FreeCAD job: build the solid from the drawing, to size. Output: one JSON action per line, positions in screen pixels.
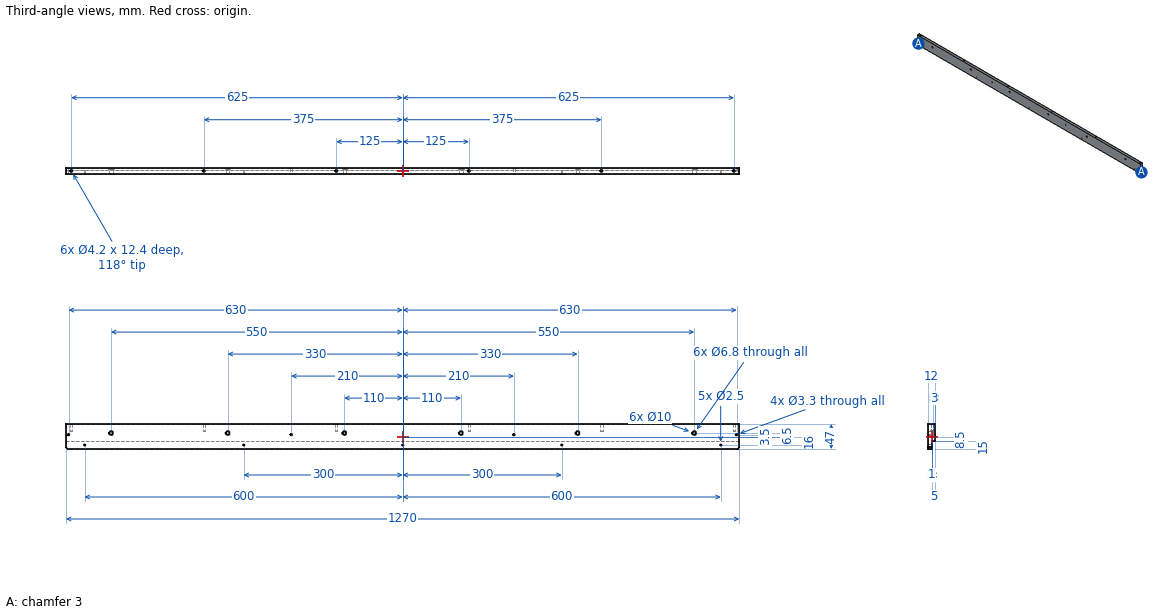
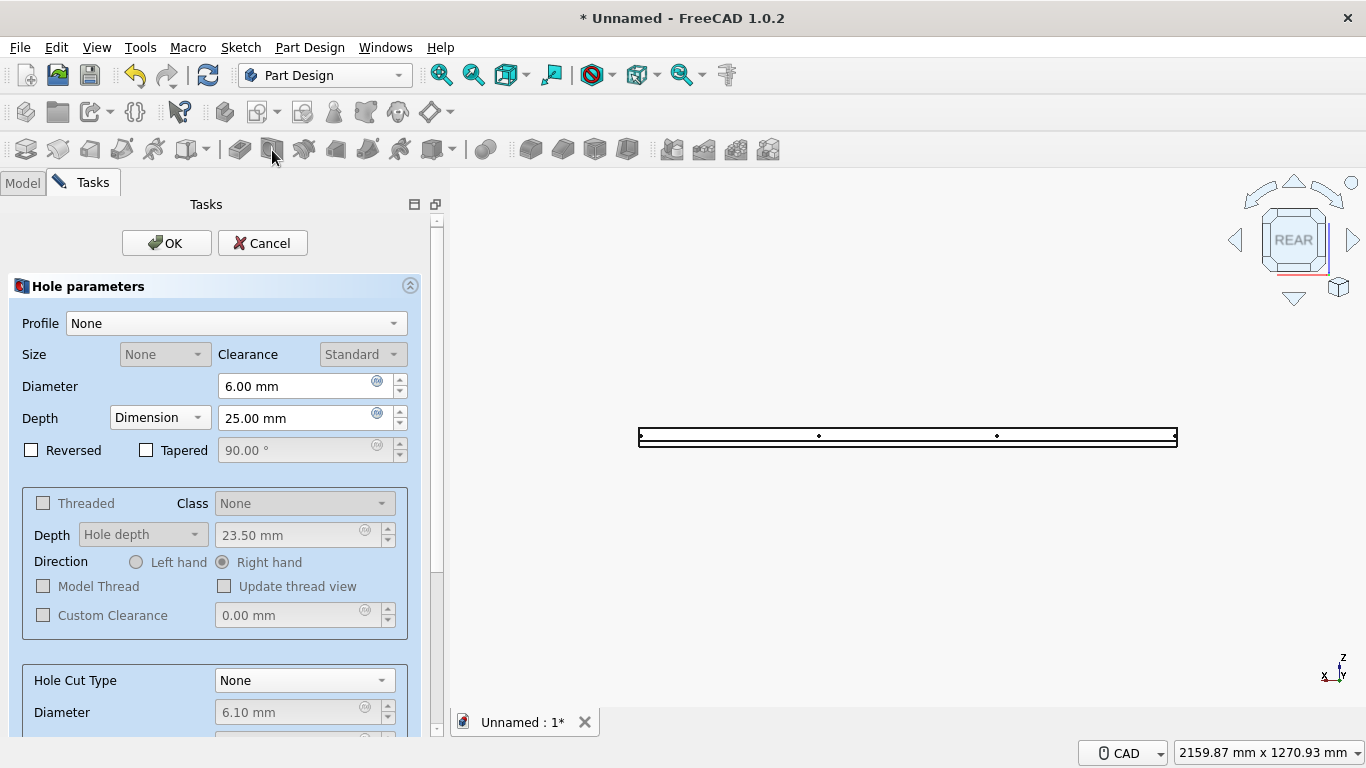
{"action": "triple_click", "coordinate": [305, 386]}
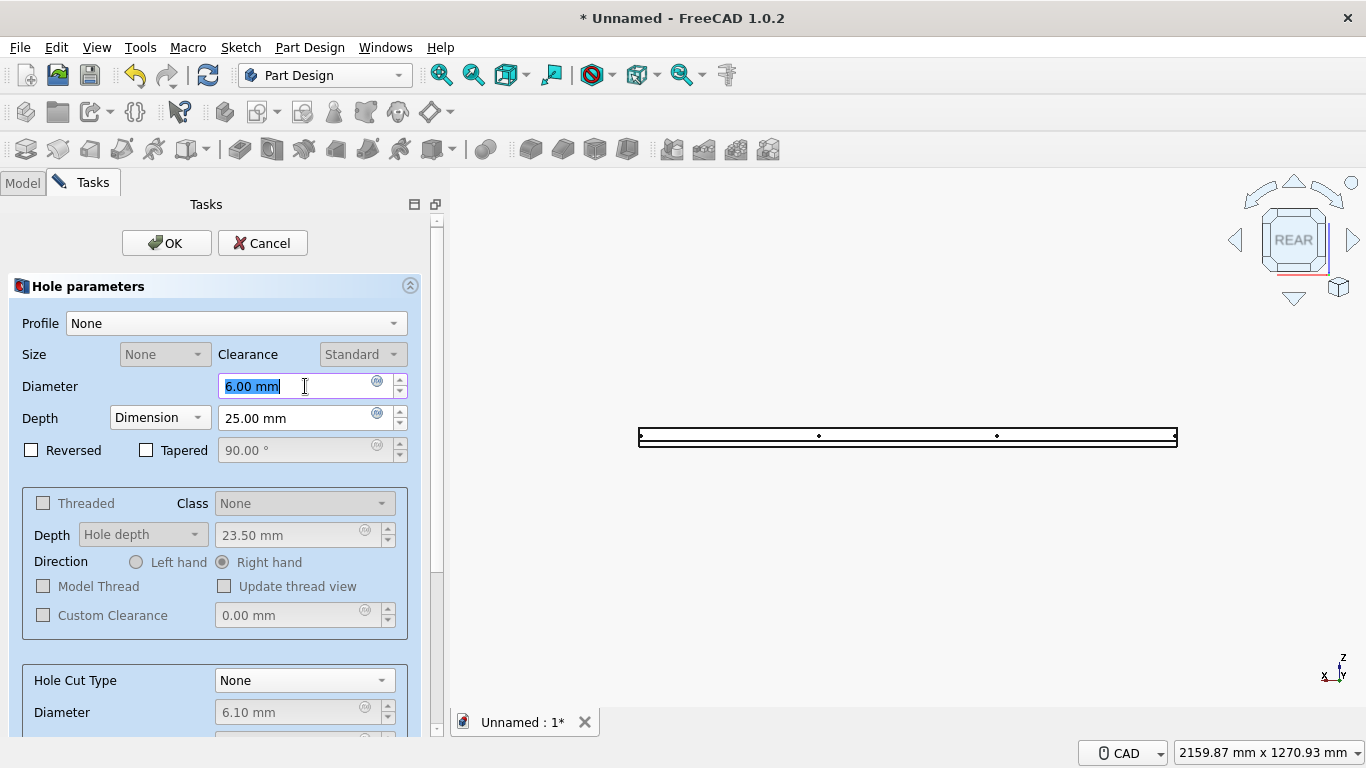
{"action": "type", "text": "3.3"}
{"action": "key", "text": "Tab"}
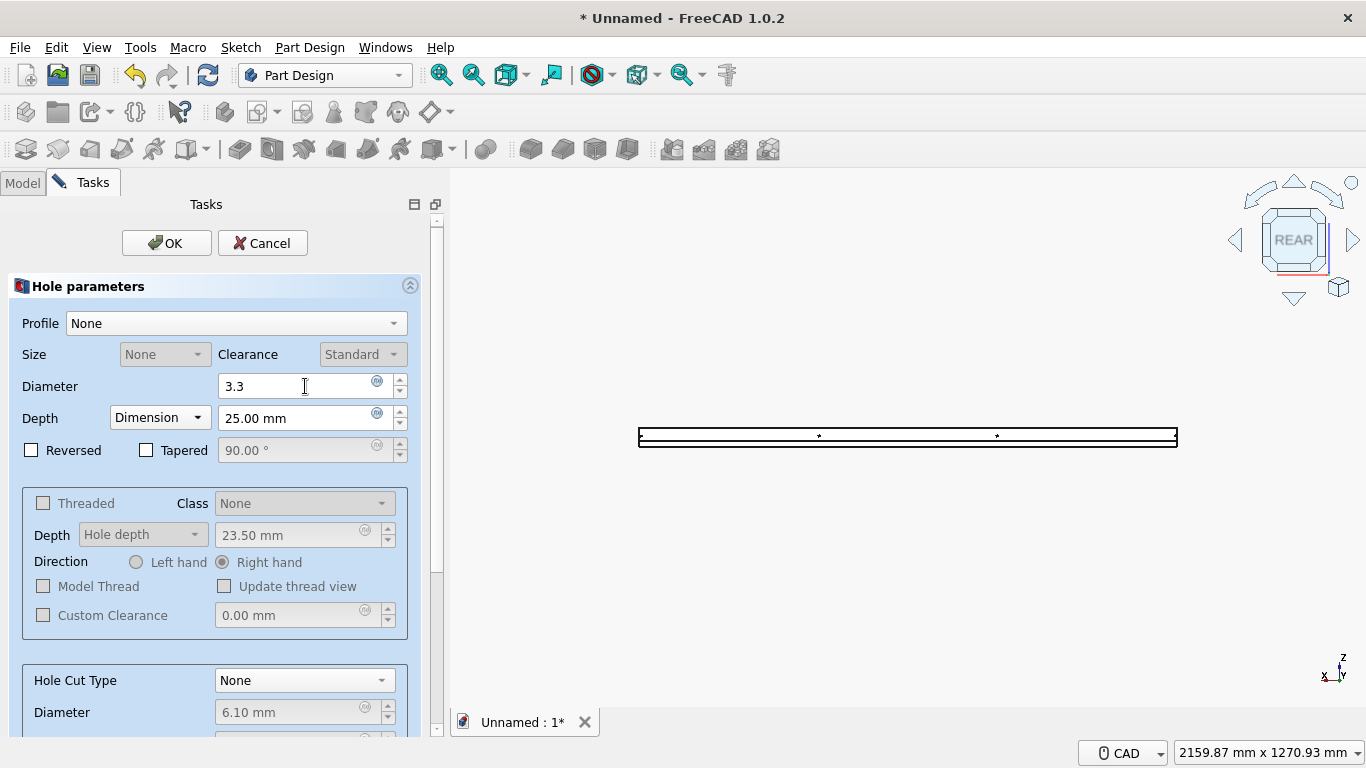
{"action": "left_click", "coordinate": [161, 418]}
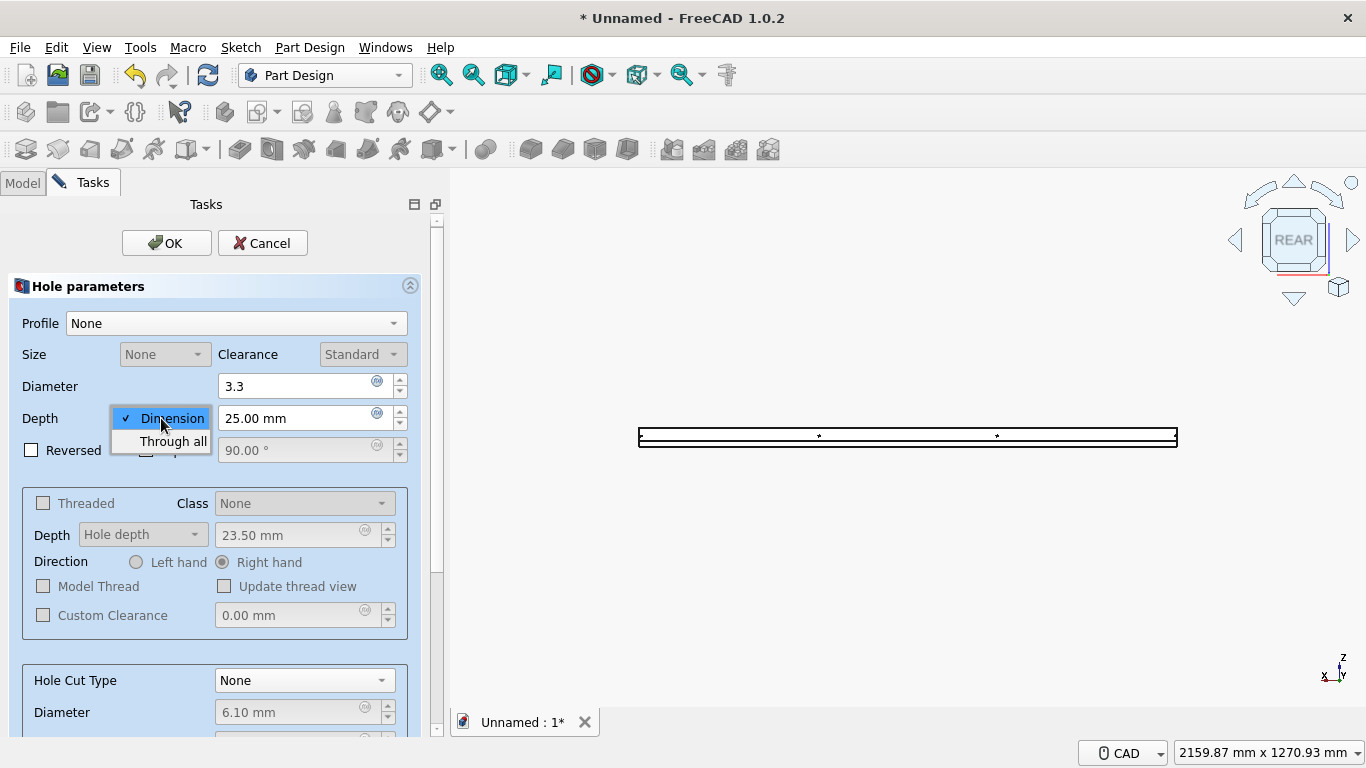
{"action": "left_click", "coordinate": [160, 442]}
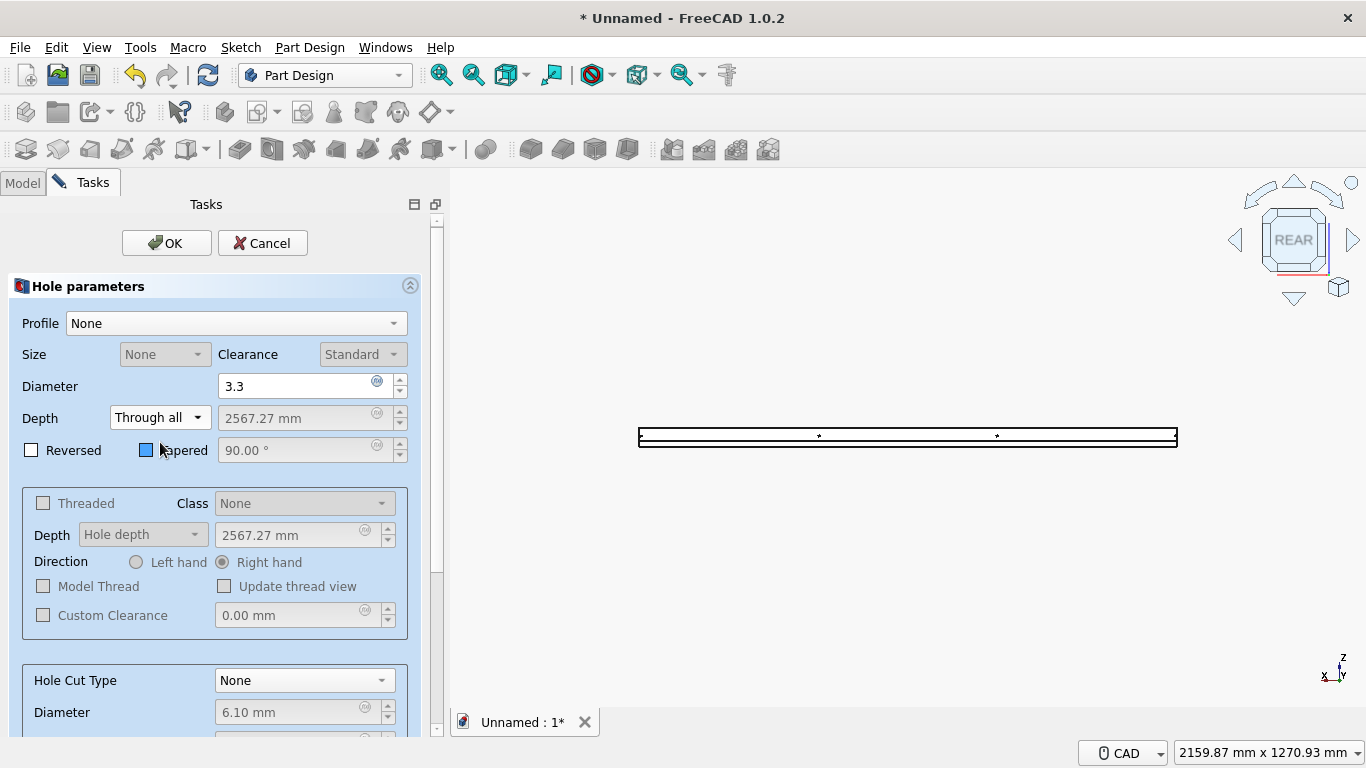
{"action": "left_click", "coordinate": [167, 243]}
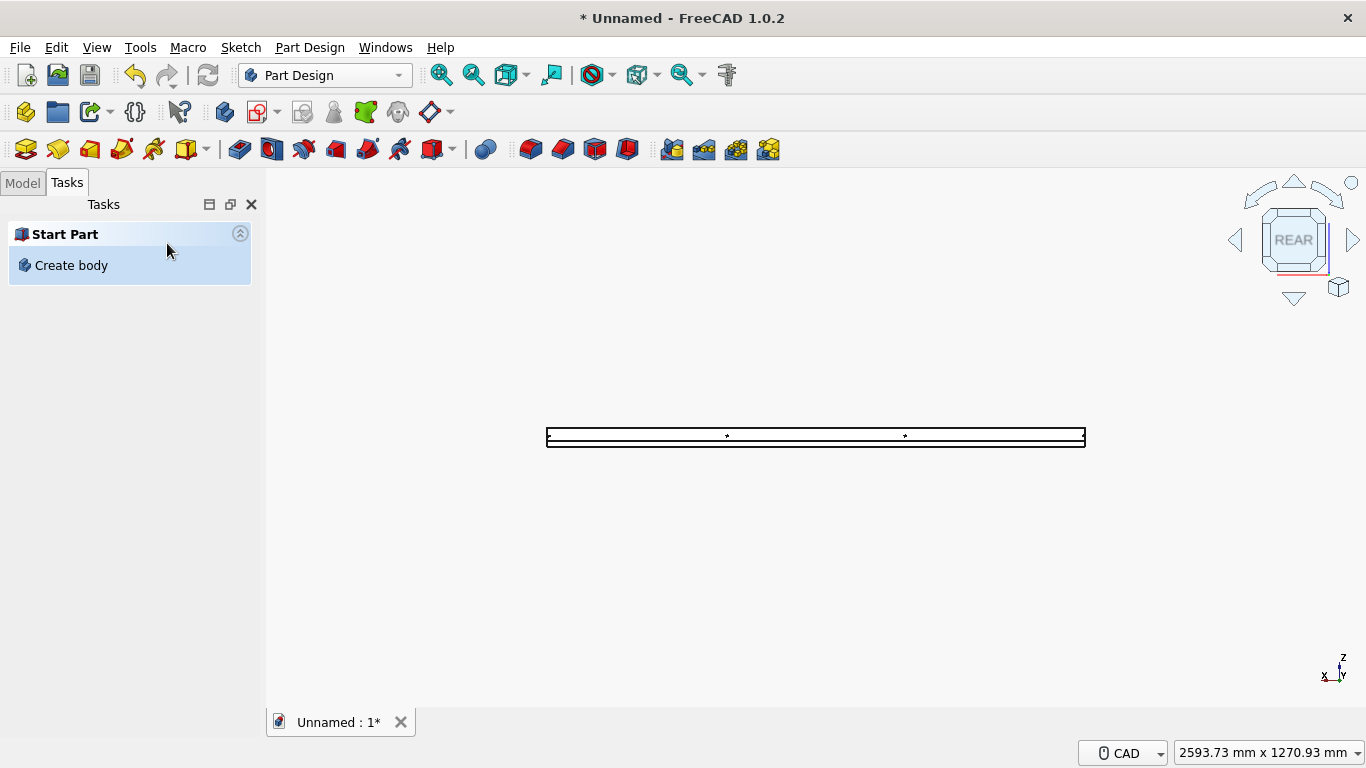
{"action": "key", "text": "0"}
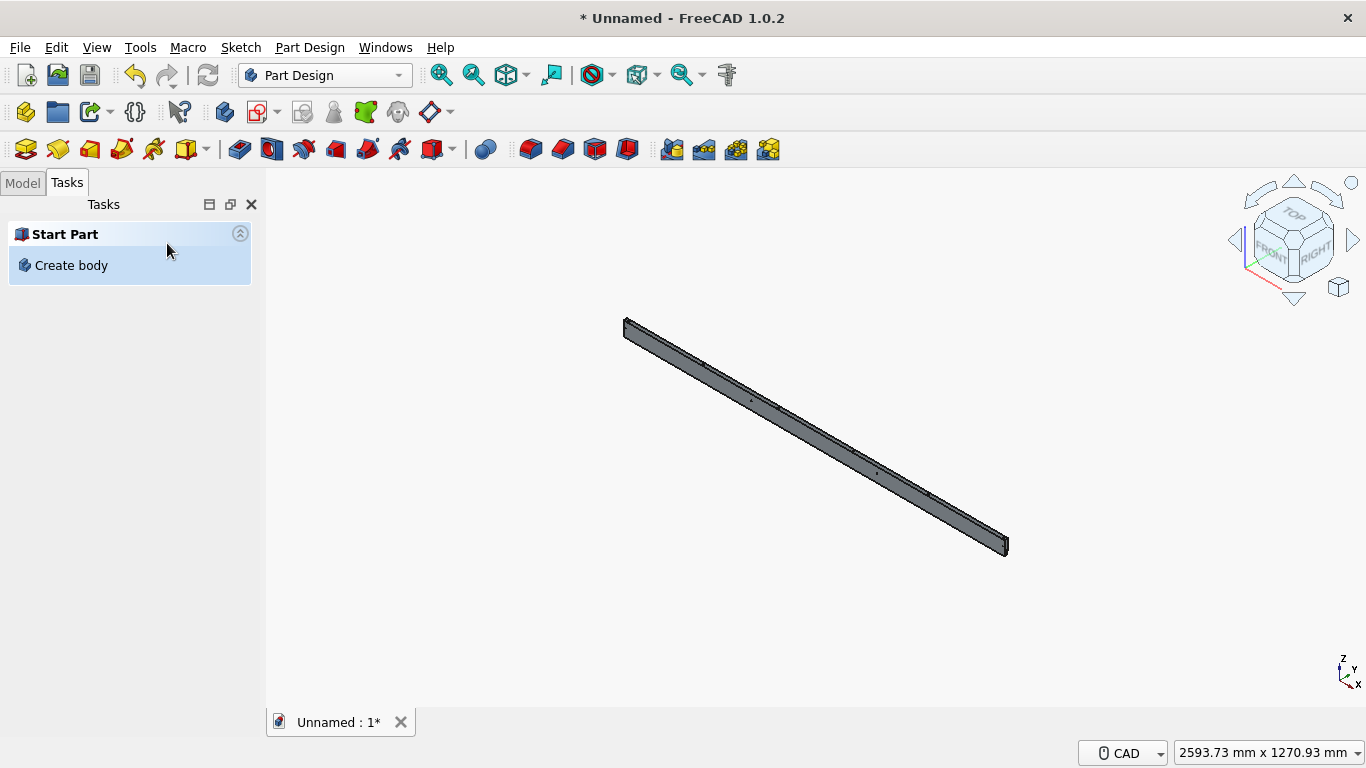
{"action": "left_click", "coordinate": [442, 76]}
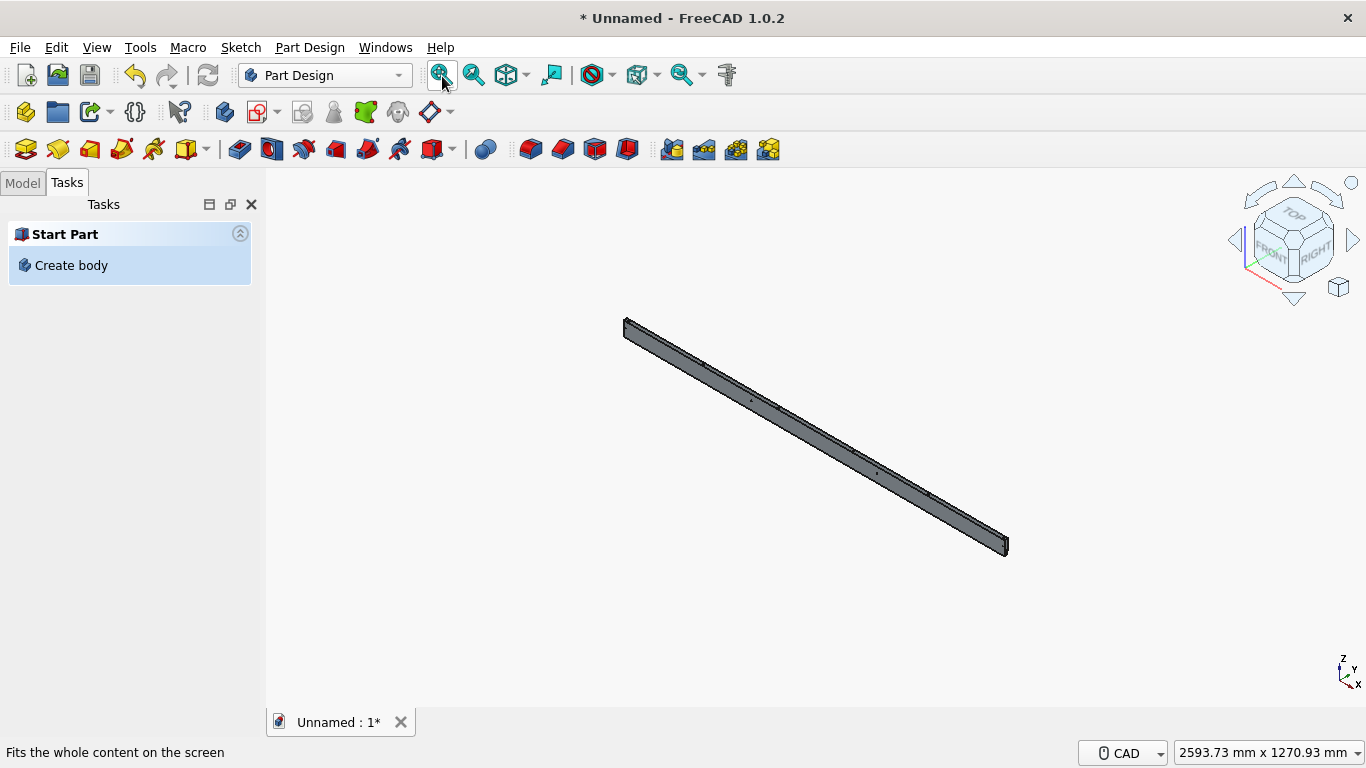
{"action": "left_click", "coordinate": [977, 534]}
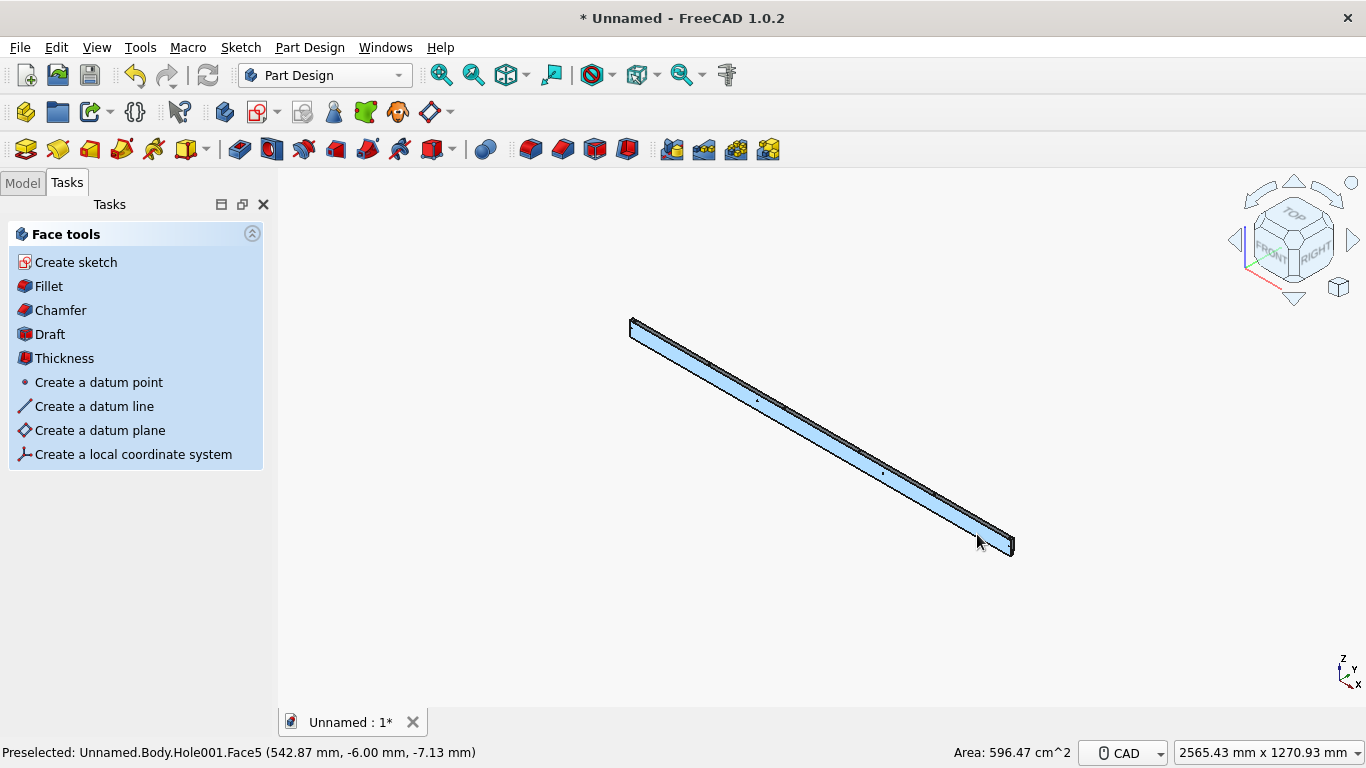
{"action": "left_click", "coordinate": [258, 112]}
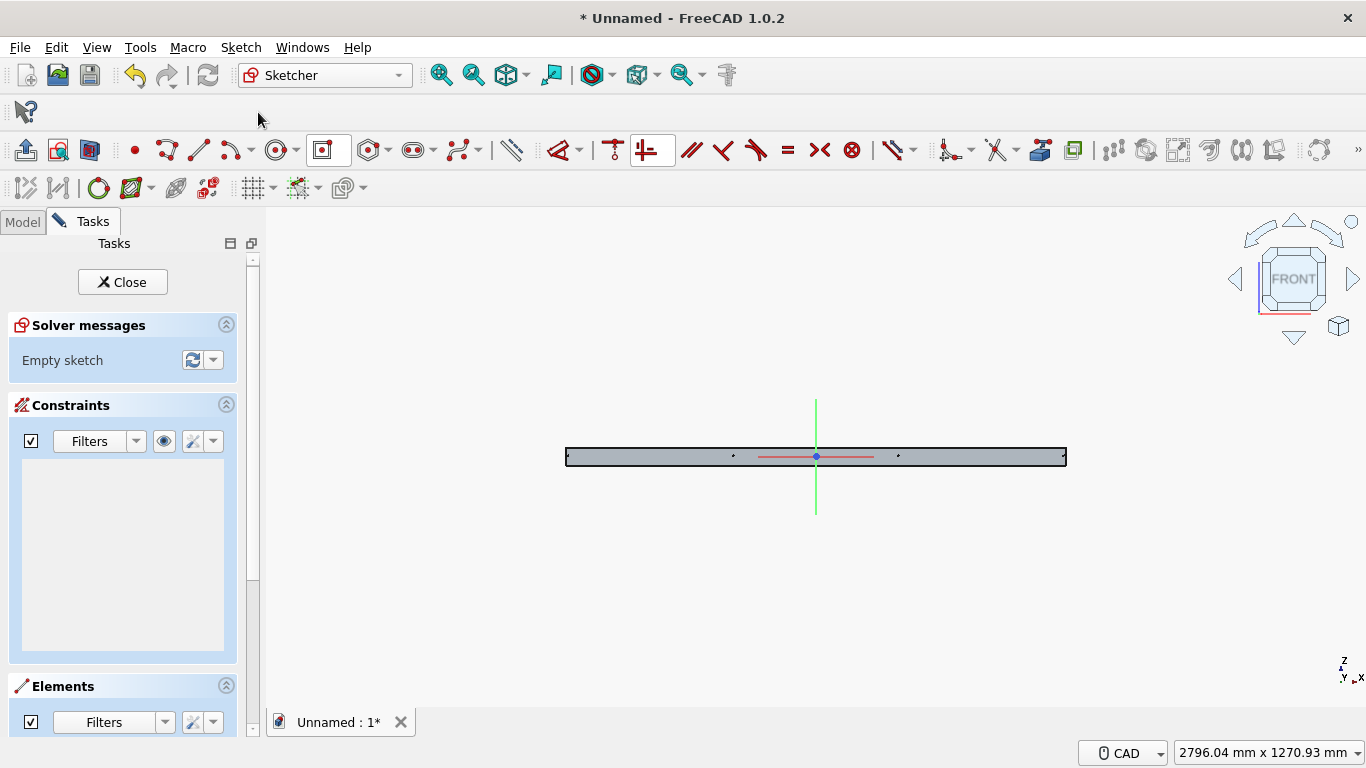
{"action": "scroll", "coordinate": [955, 467], "scroll_direction": "up", "scroll_amount": 2}